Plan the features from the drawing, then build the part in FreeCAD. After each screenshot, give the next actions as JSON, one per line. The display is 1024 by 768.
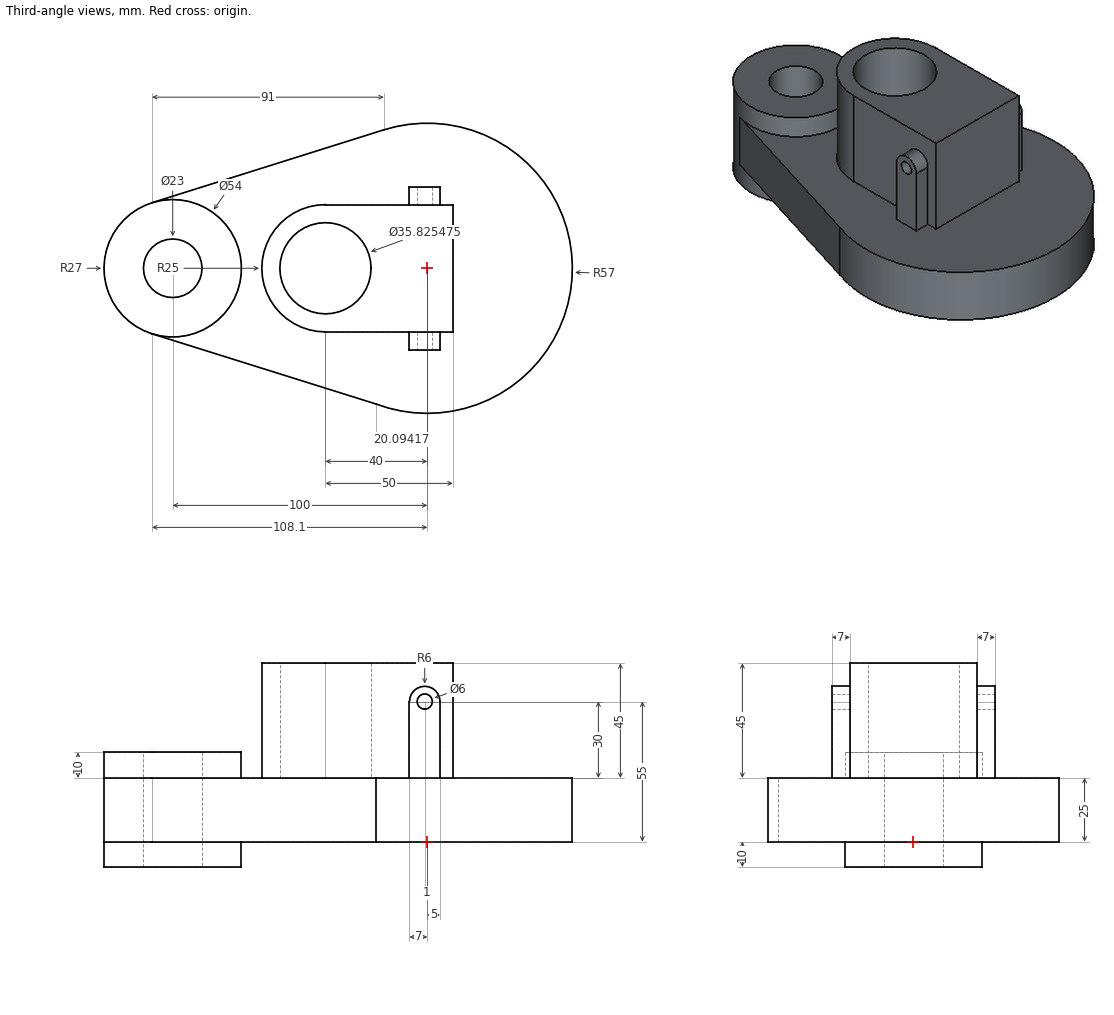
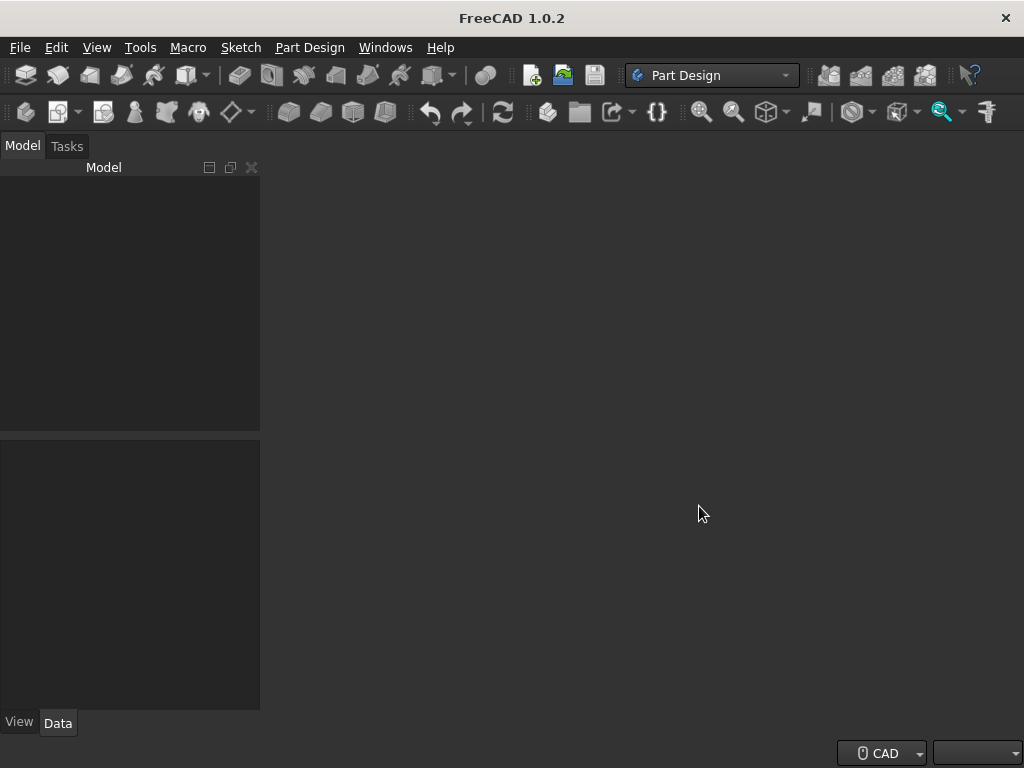
{"action": "left_click", "coordinate": [532, 76]}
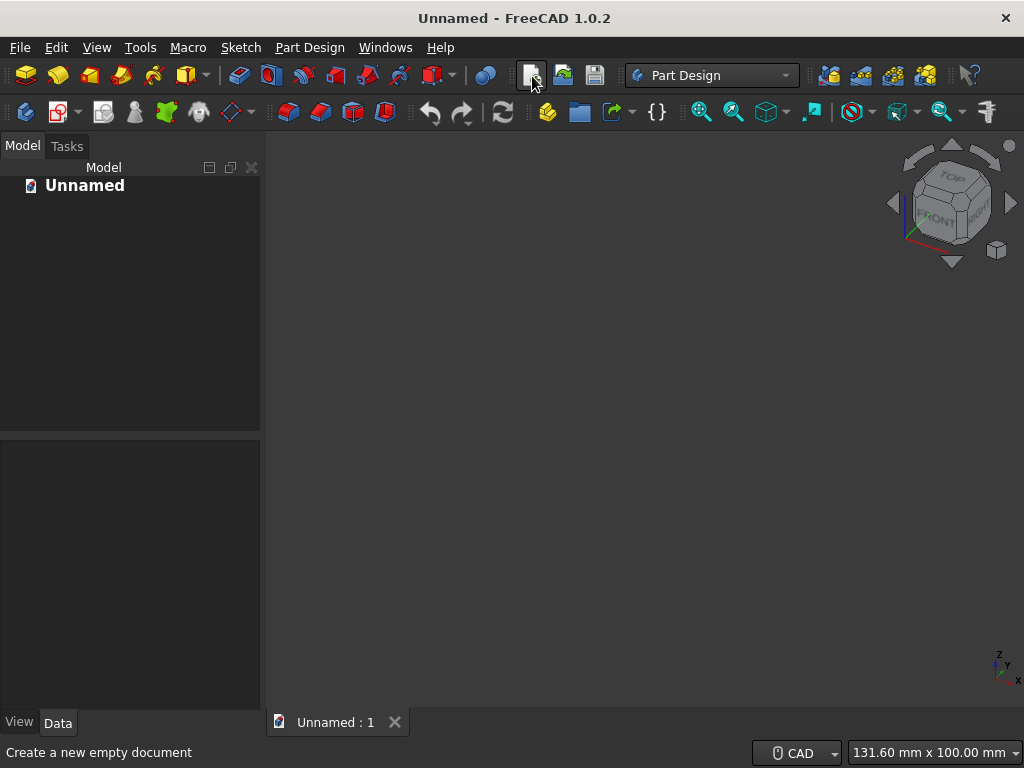
{"action": "left_click", "coordinate": [58, 112]}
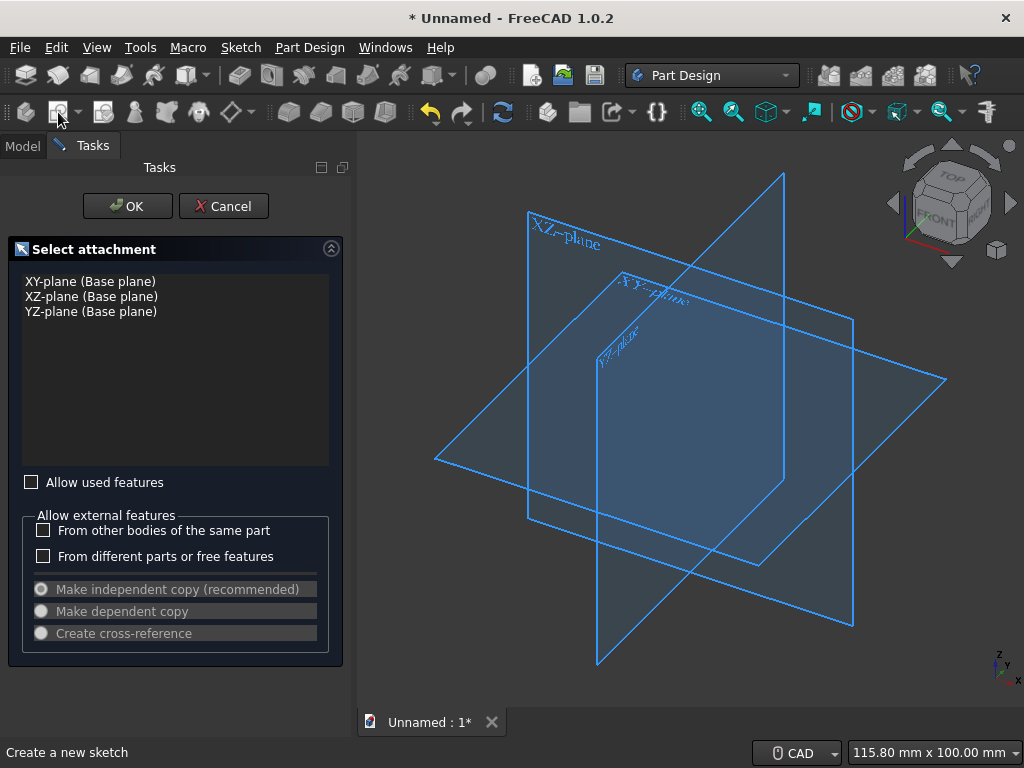
{"action": "left_click", "coordinate": [82, 282]}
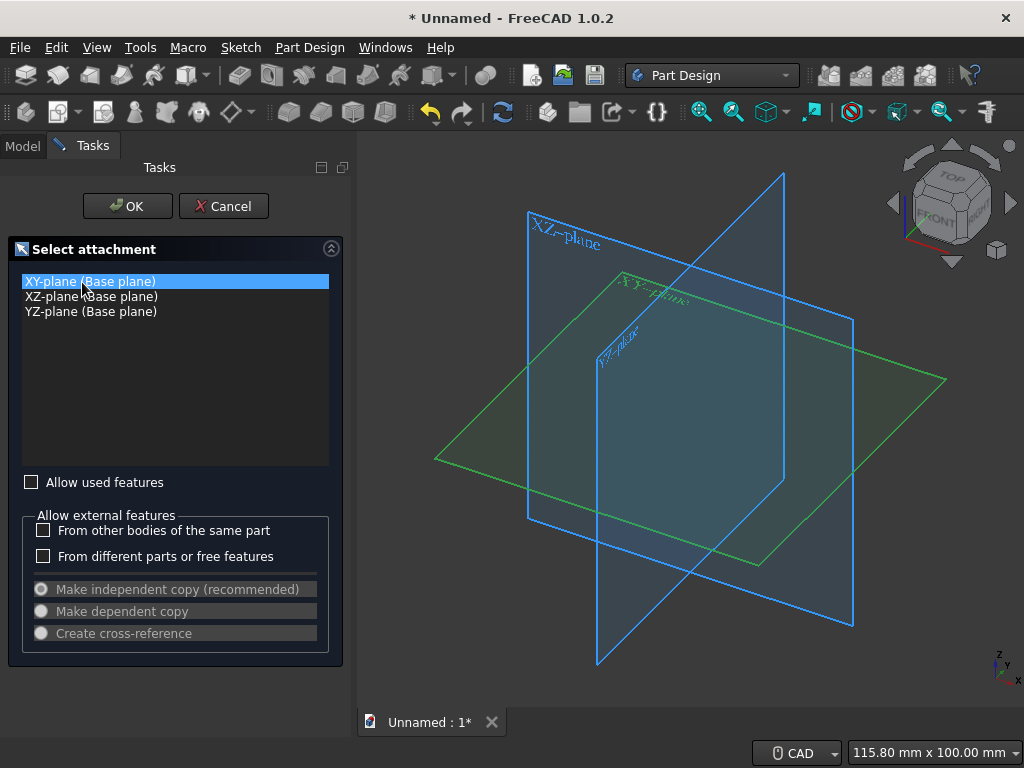
{"action": "left_click", "coordinate": [128, 206]}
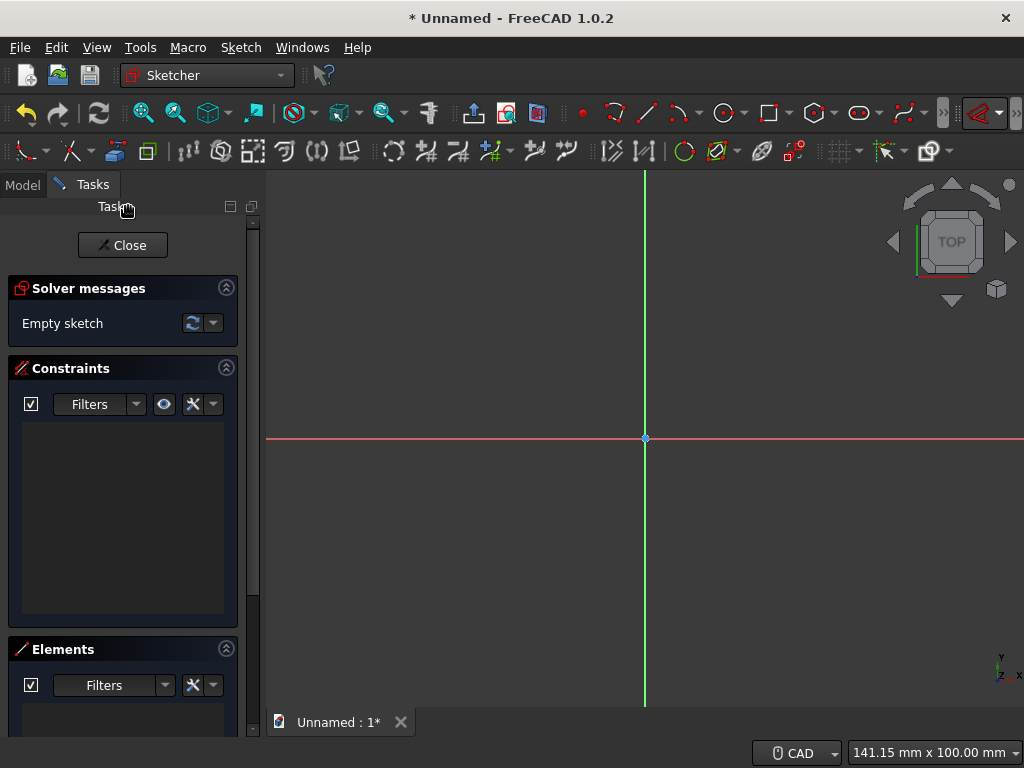
{"action": "scroll", "coordinate": [646, 440], "scroll_direction": "down", "scroll_amount": 5}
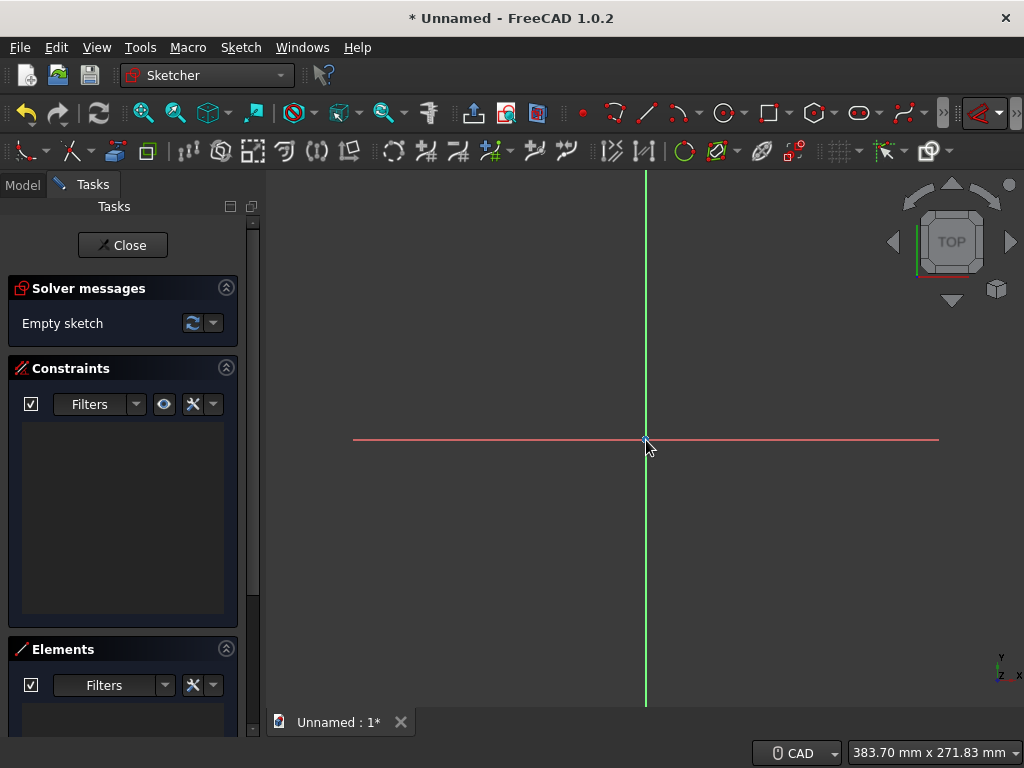
{"action": "key", "text": "g l"}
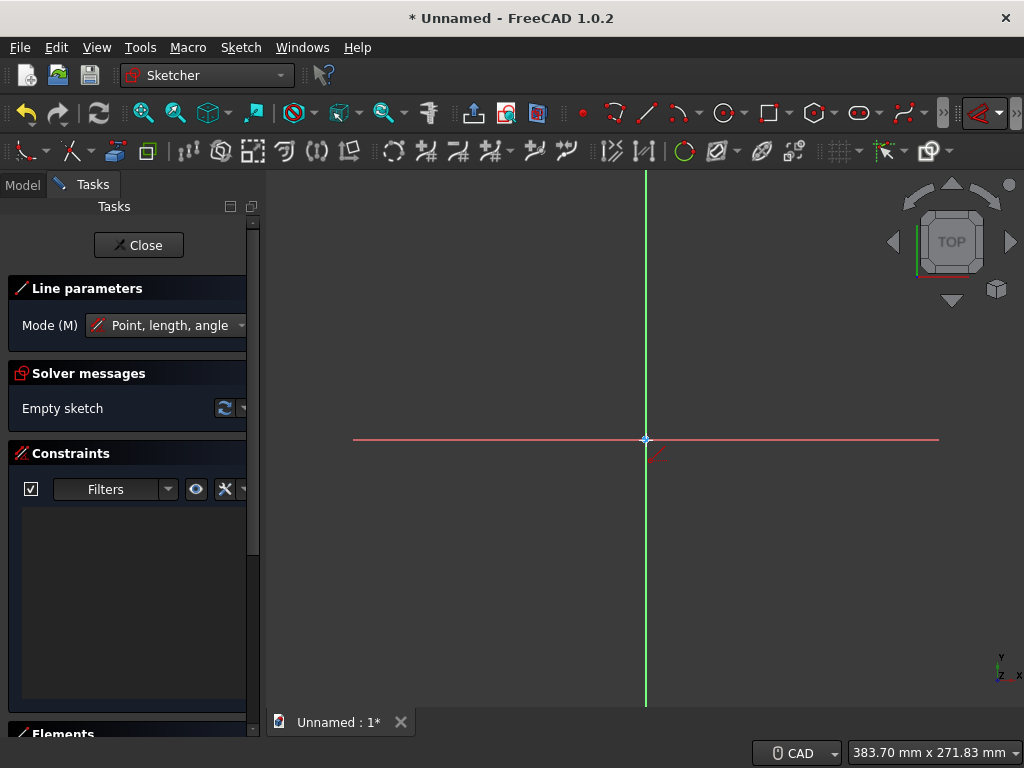
{"action": "left_click", "coordinate": [612, 332]}
{"action": "left_click", "coordinate": [432, 389]}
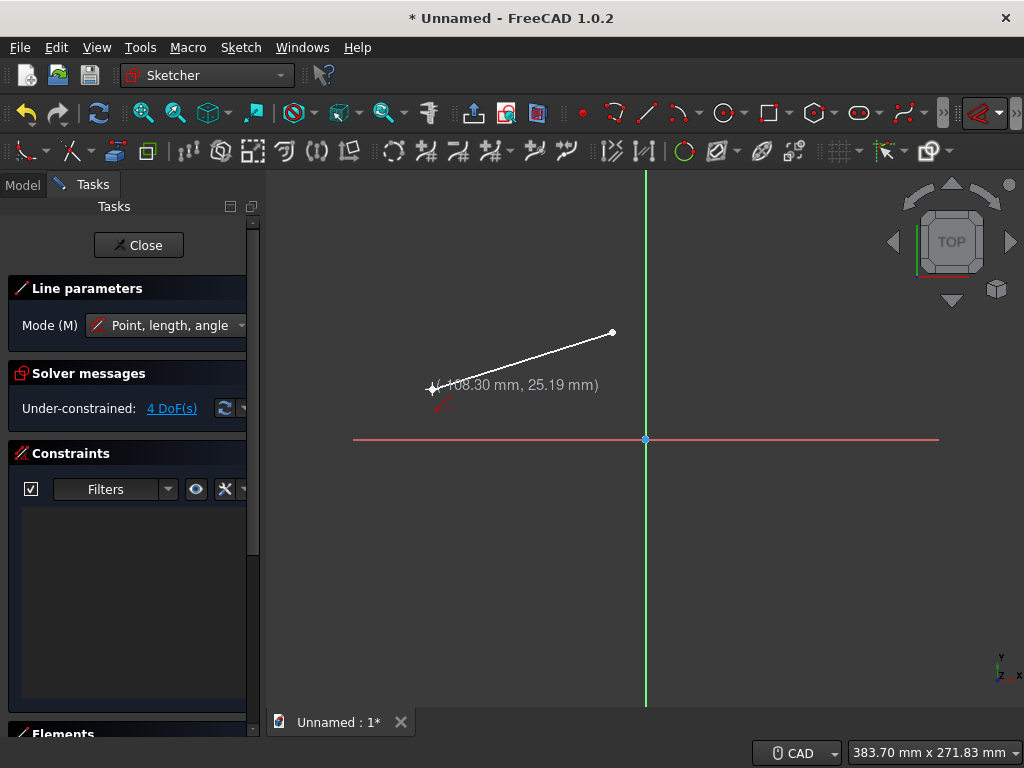
{"action": "left_click", "coordinate": [432, 491]}
{"action": "left_click", "coordinate": [606, 545]}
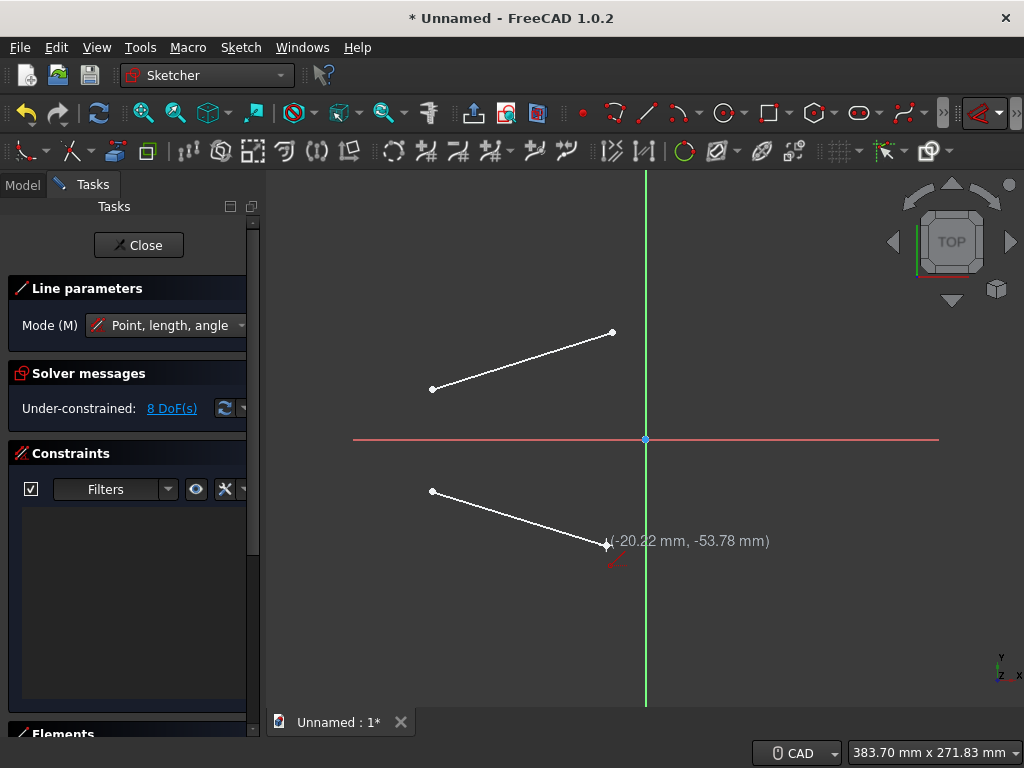
{"action": "key", "text": "g 3 a"}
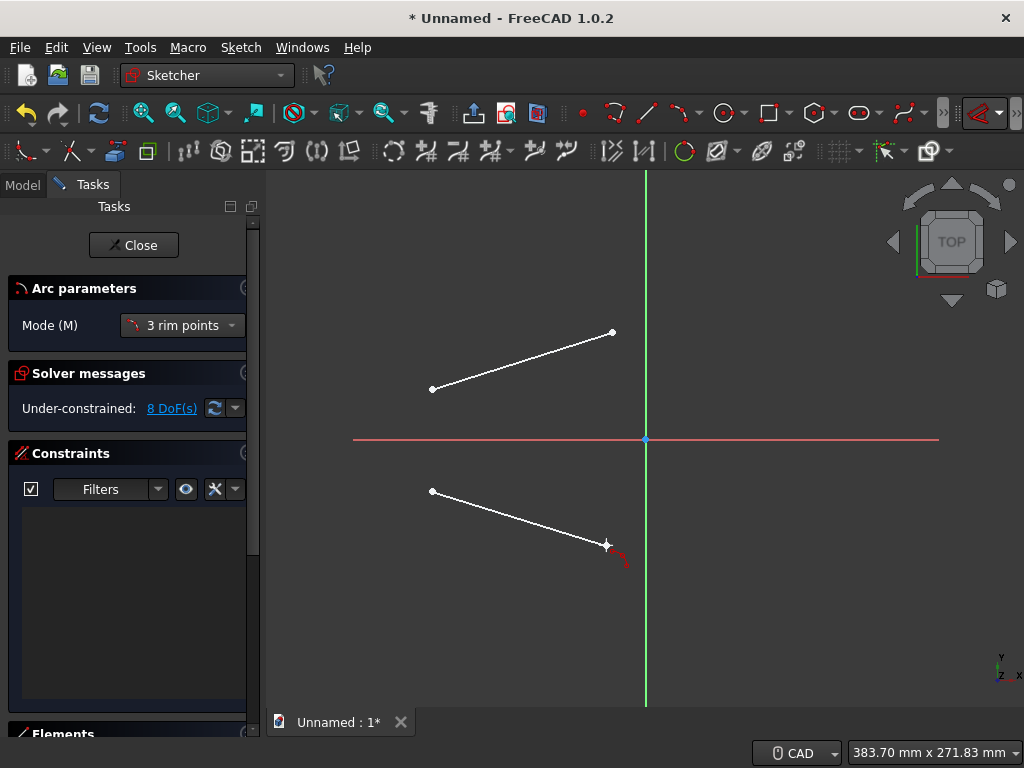
{"action": "left_click", "coordinate": [432, 390]}
{"action": "left_click", "coordinate": [432, 492]}
{"action": "left_click", "coordinate": [402, 414]}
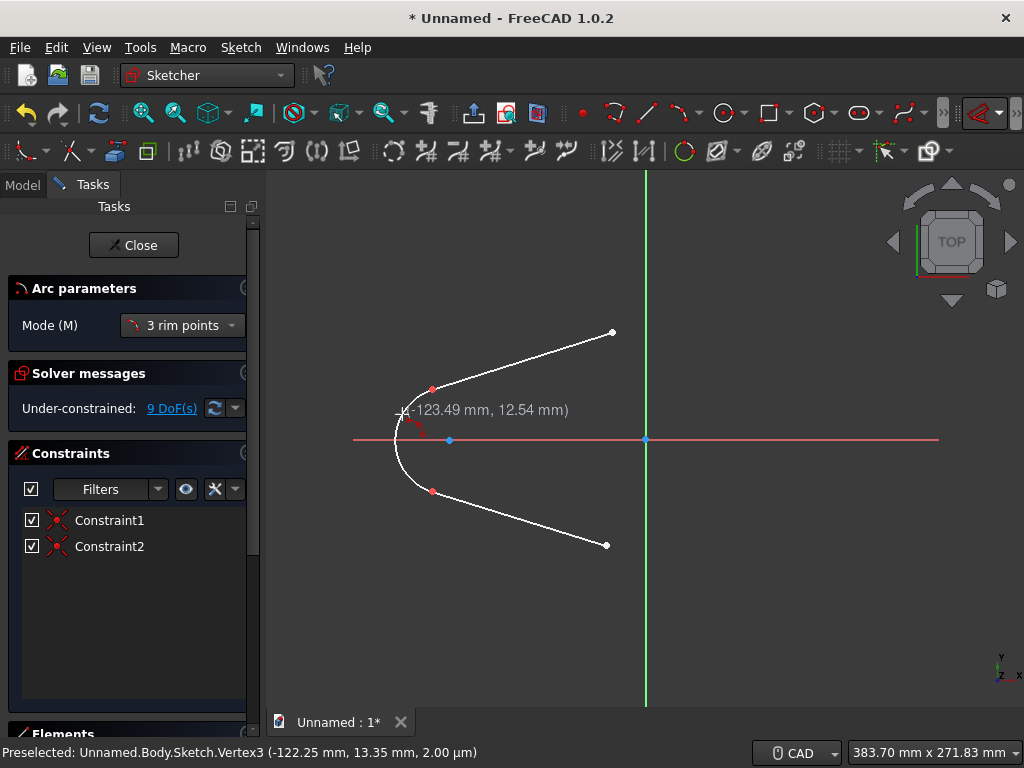
{"action": "left_click", "coordinate": [606, 546]}
{"action": "left_click", "coordinate": [612, 333]}
{"action": "left_click", "coordinate": [749, 484]}
{"action": "key", "text": "Escape"}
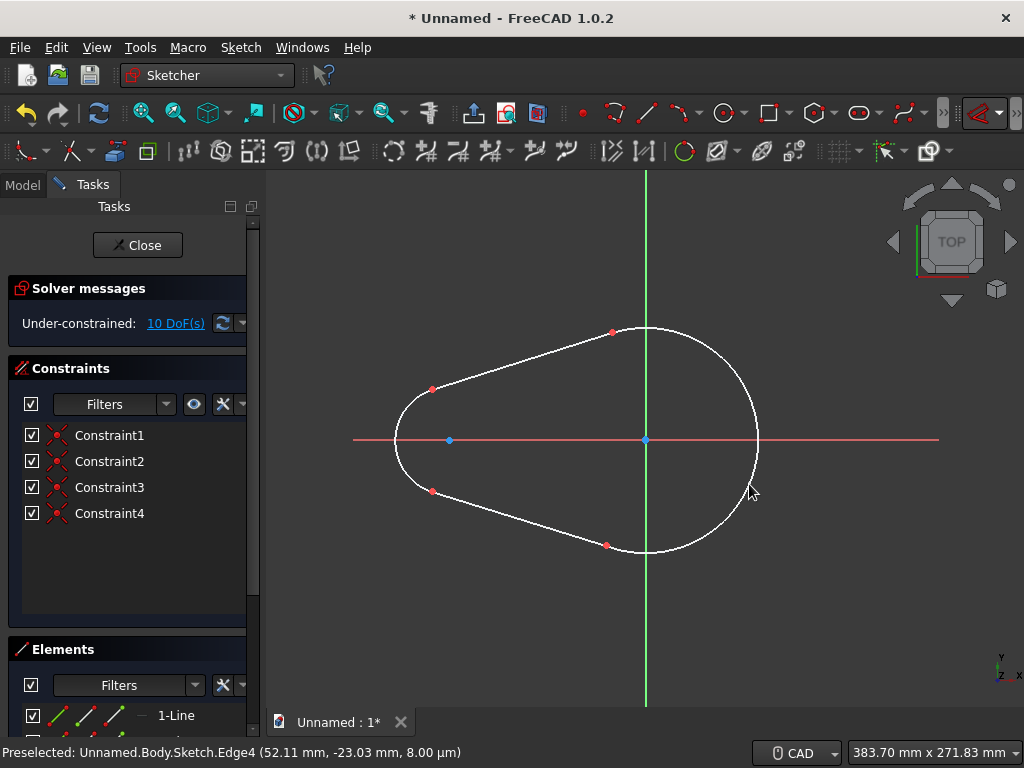
{"action": "left_click", "coordinate": [558, 350]}